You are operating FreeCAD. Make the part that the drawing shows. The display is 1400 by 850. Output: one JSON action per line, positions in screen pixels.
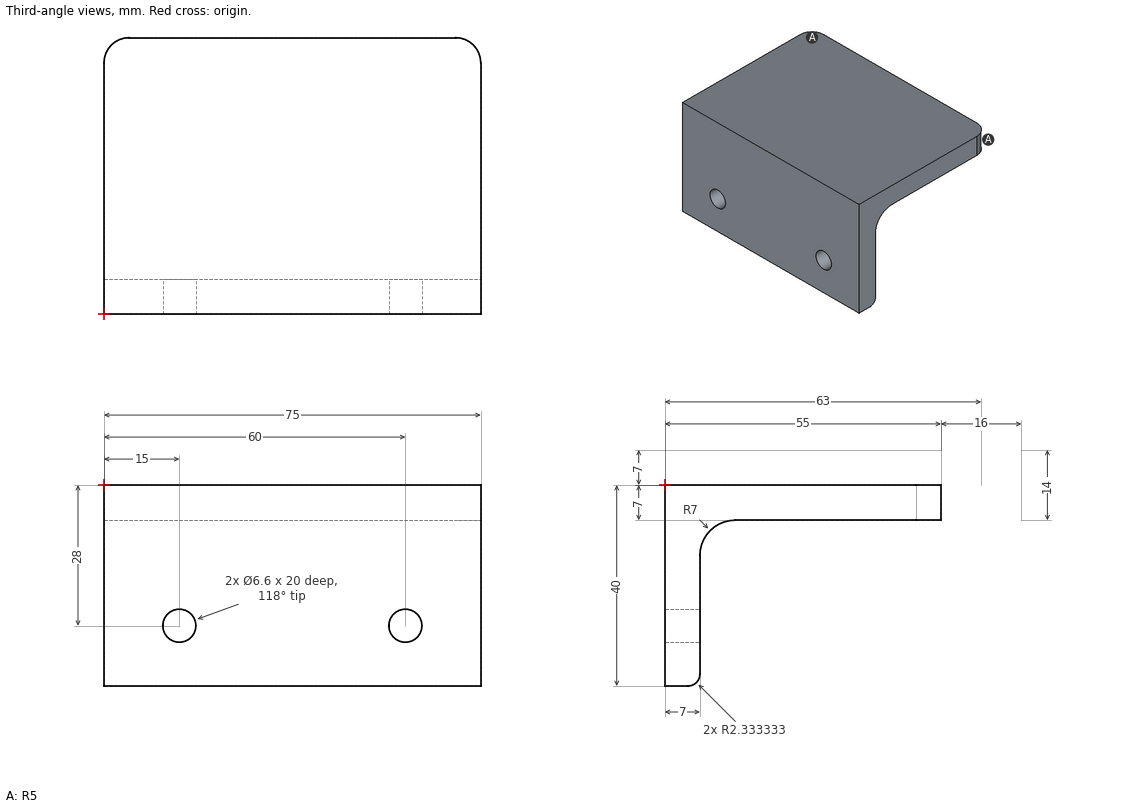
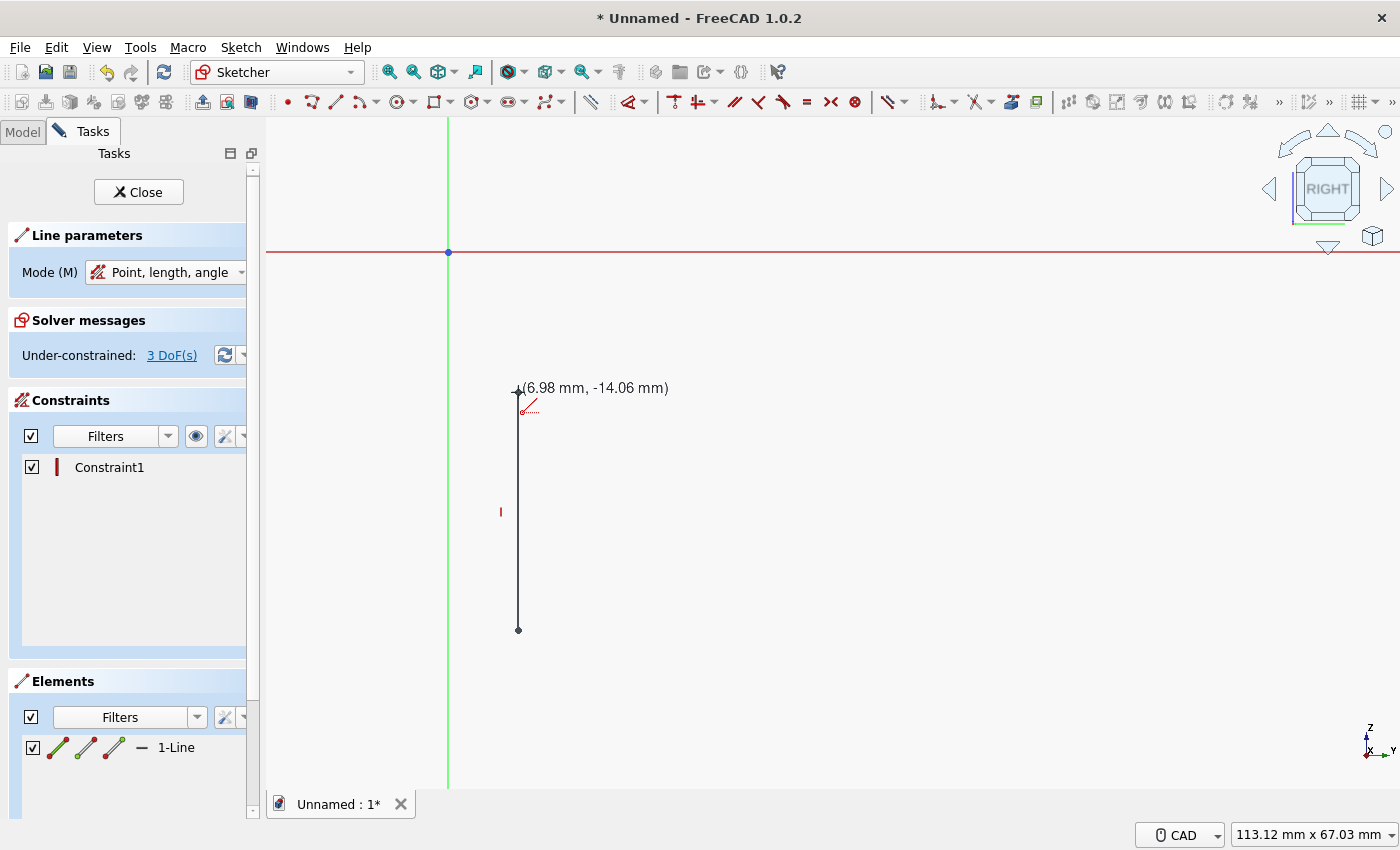
{"action": "left_click", "coordinate": [588, 322]}
{"action": "left_click", "coordinate": [1056, 322]}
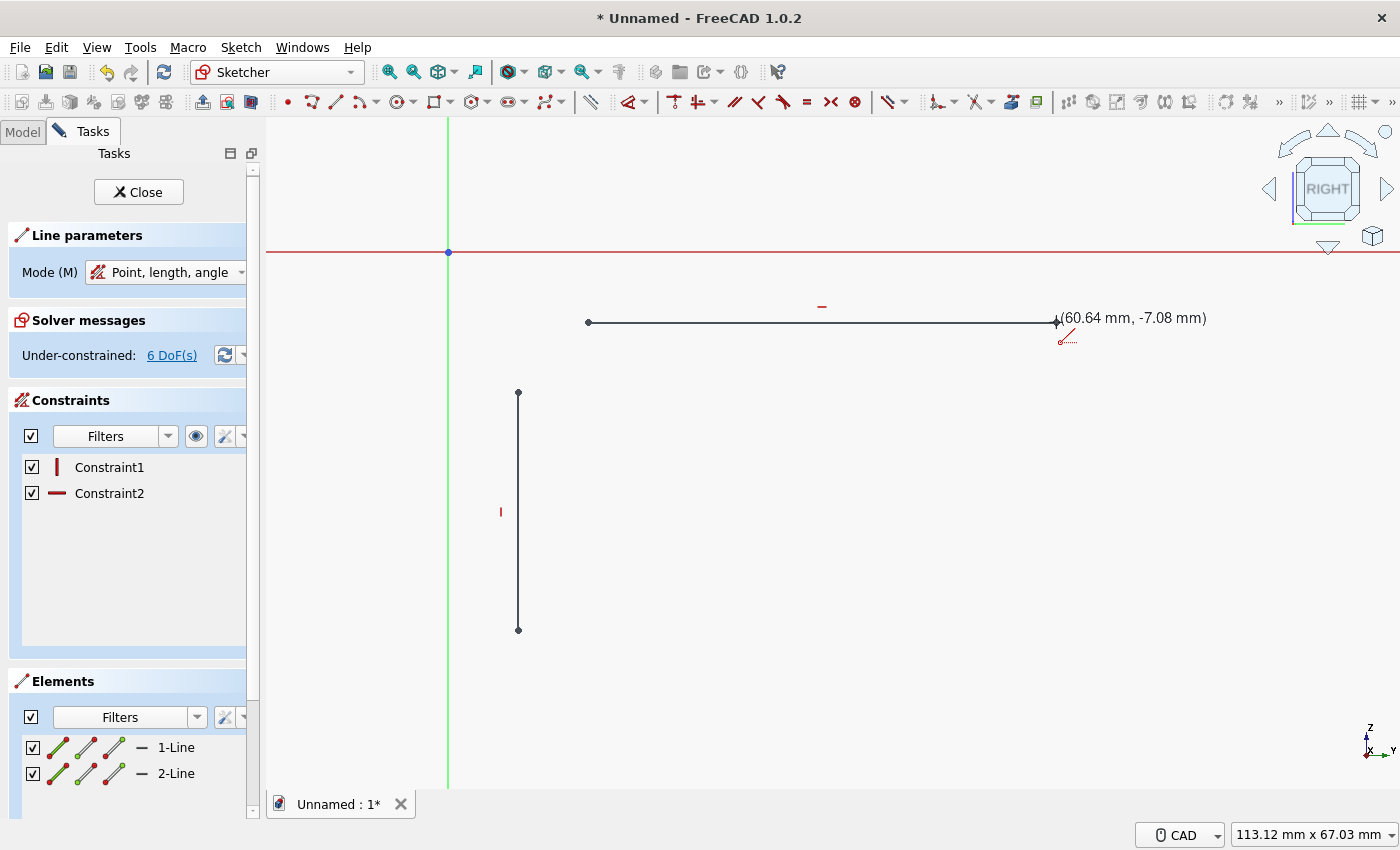
{"action": "left_click", "coordinate": [312, 102]}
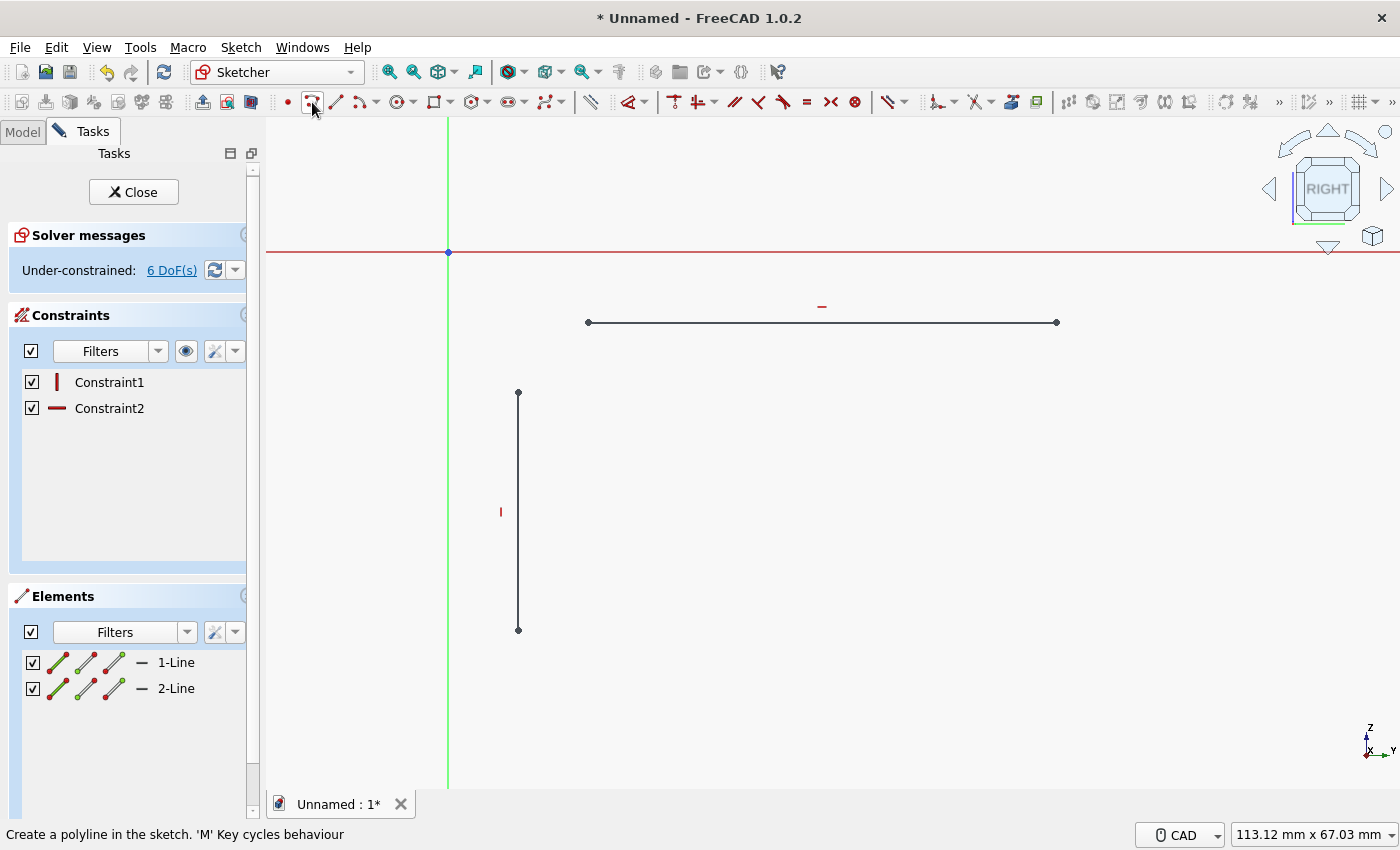
{"action": "left_click", "coordinate": [1080, 299]}
{"action": "left_click", "coordinate": [1080, 252]}
{"action": "left_click", "coordinate": [448, 252]}
{"action": "left_click", "coordinate": [457, 653]}
{"action": "left_click", "coordinate": [495, 653]}
{"action": "right_click", "coordinate": [495, 653]}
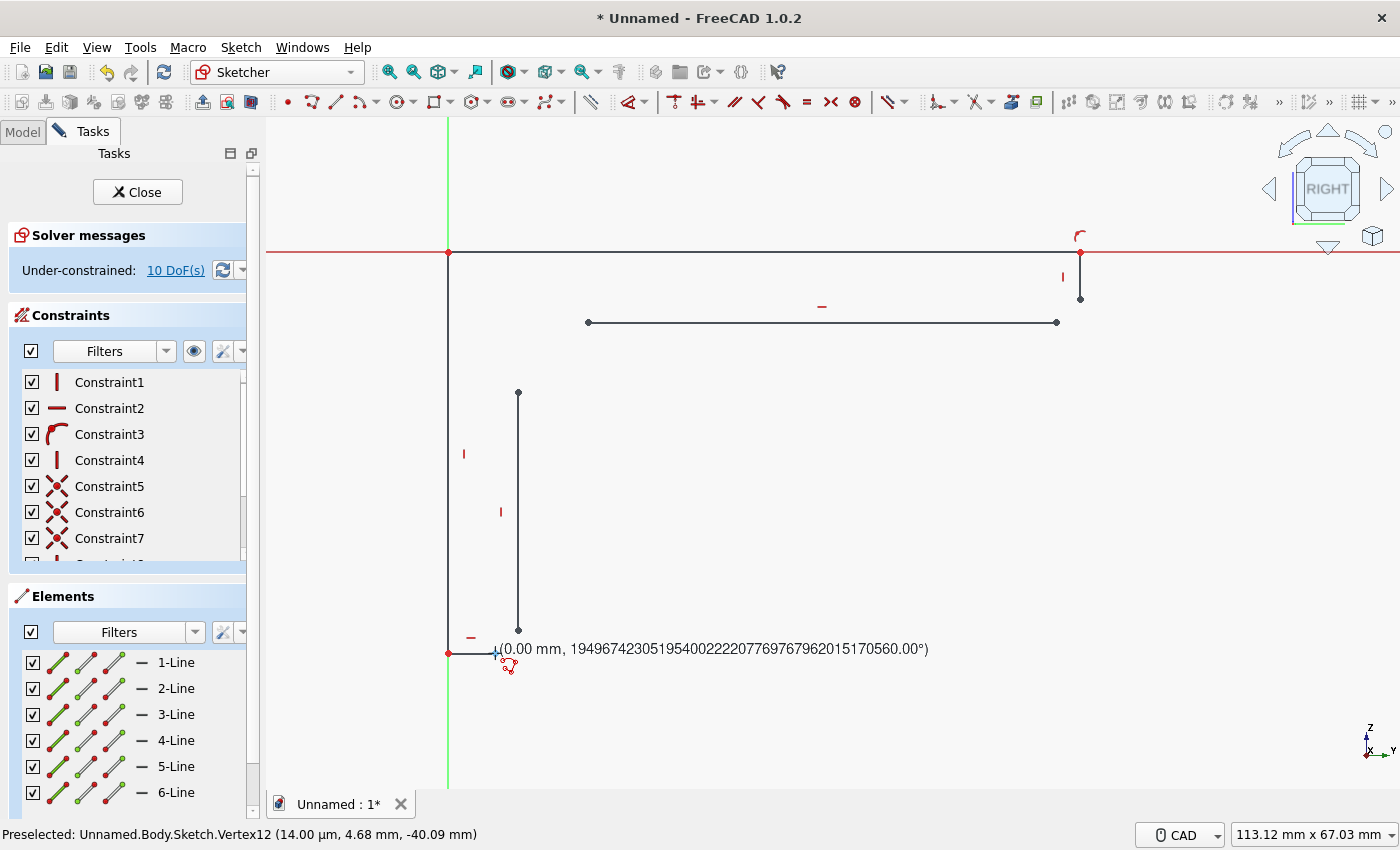
{"action": "left_click", "coordinate": [378, 102]}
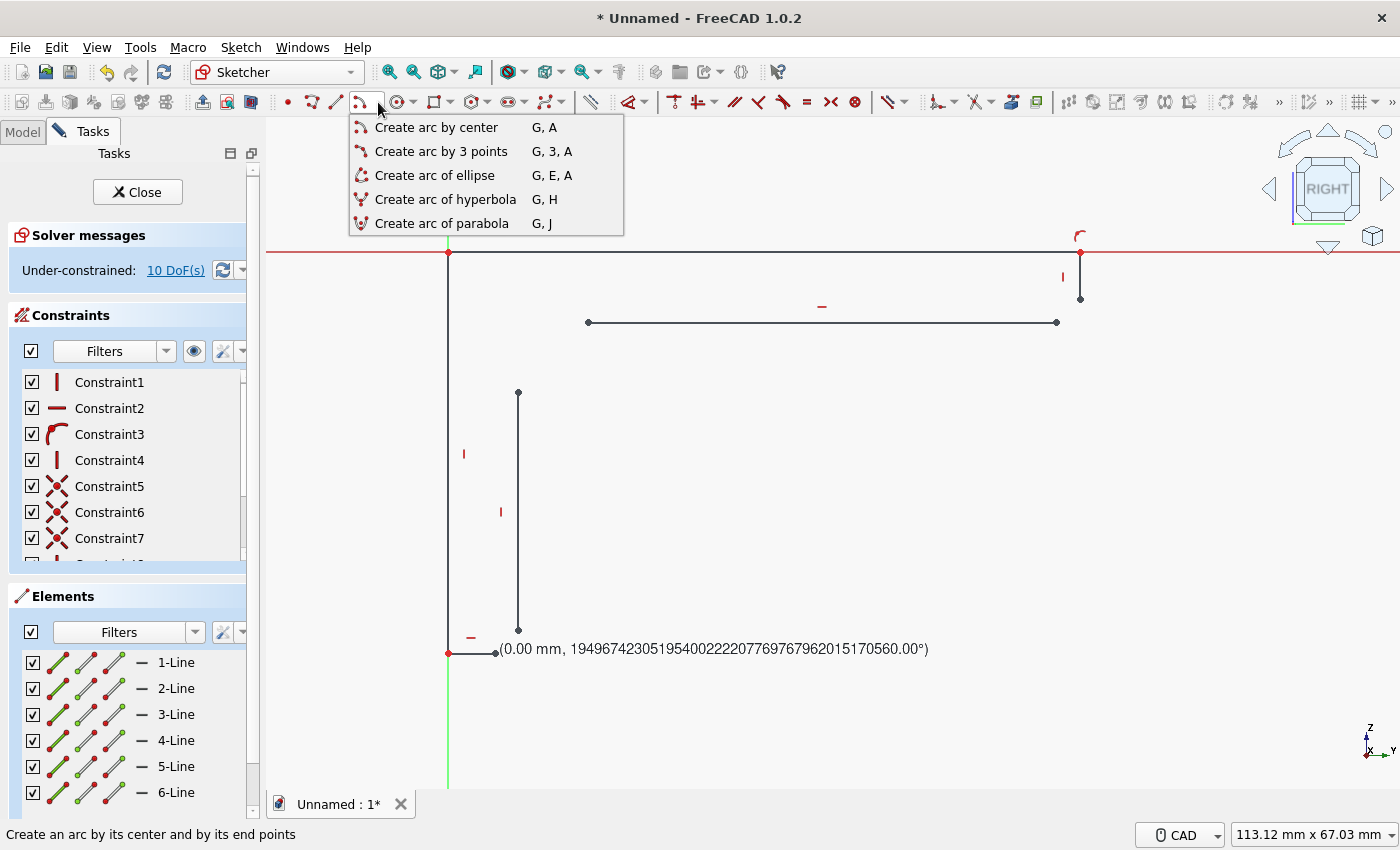
{"action": "left_click", "coordinate": [486, 151]}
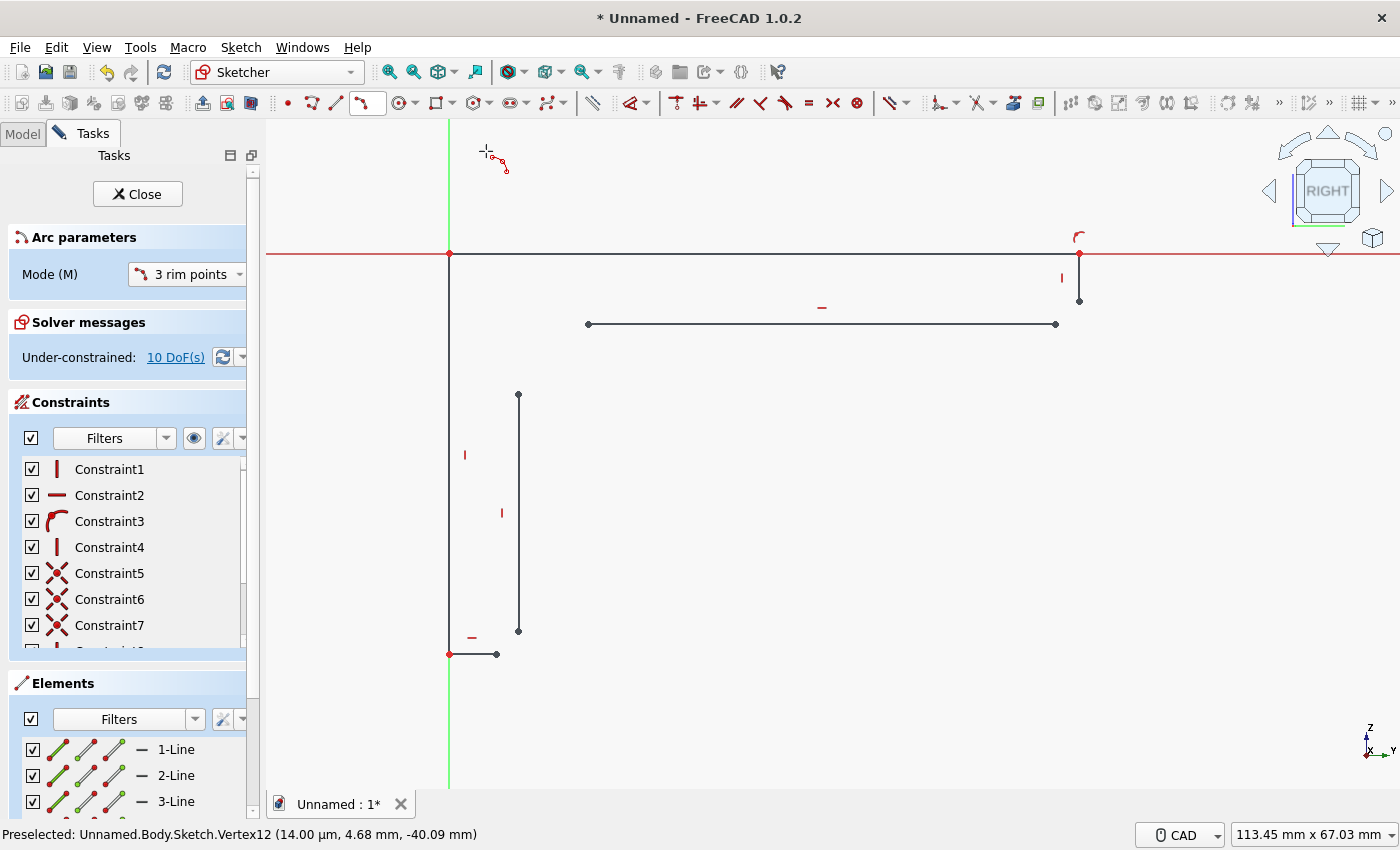
{"action": "left_click", "coordinate": [519, 394]}
{"action": "left_click", "coordinate": [589, 324]}
{"action": "left_click", "coordinate": [540, 344]}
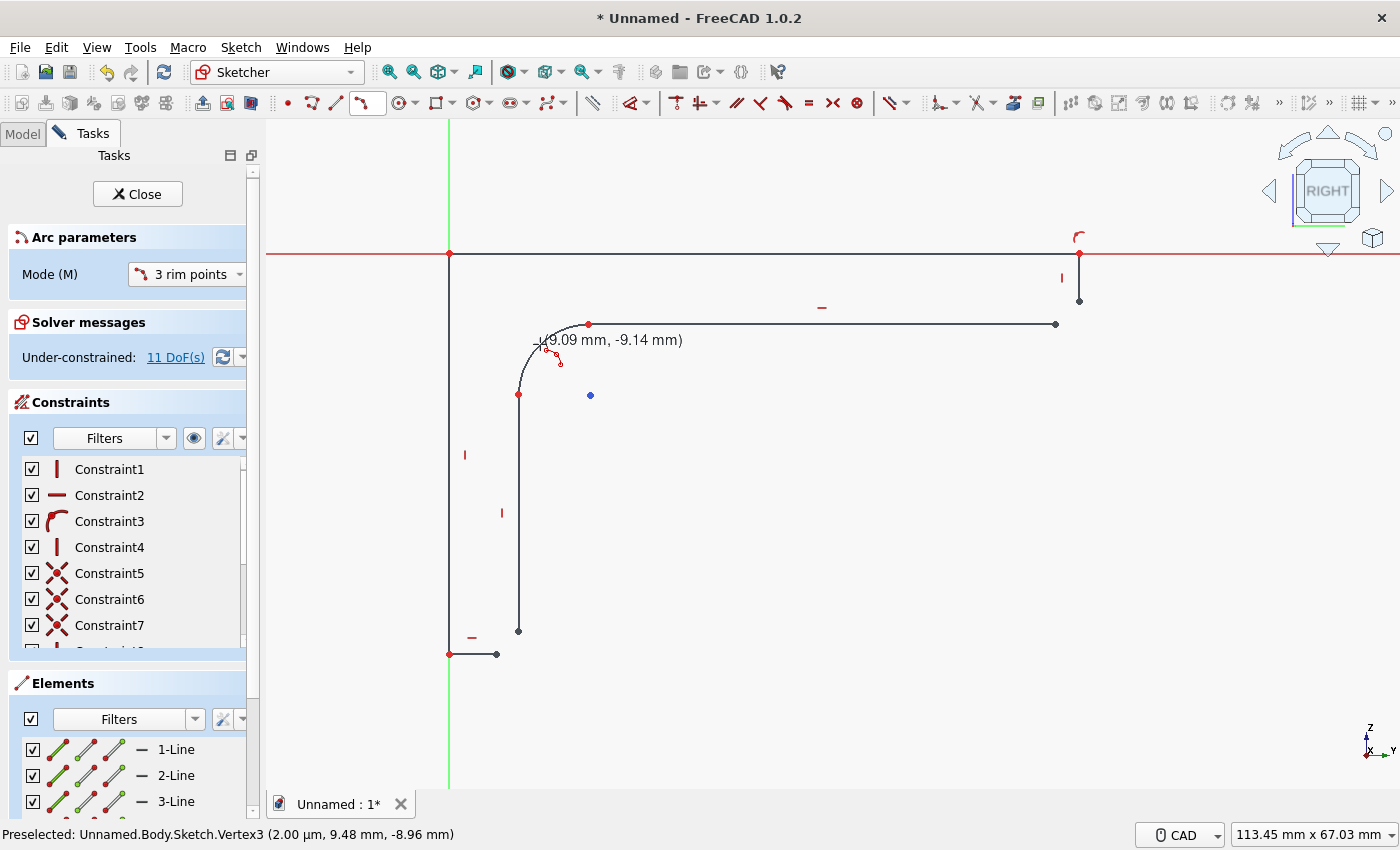
{"action": "left_click", "coordinate": [1055, 324]}
{"action": "left_click", "coordinate": [1079, 301]}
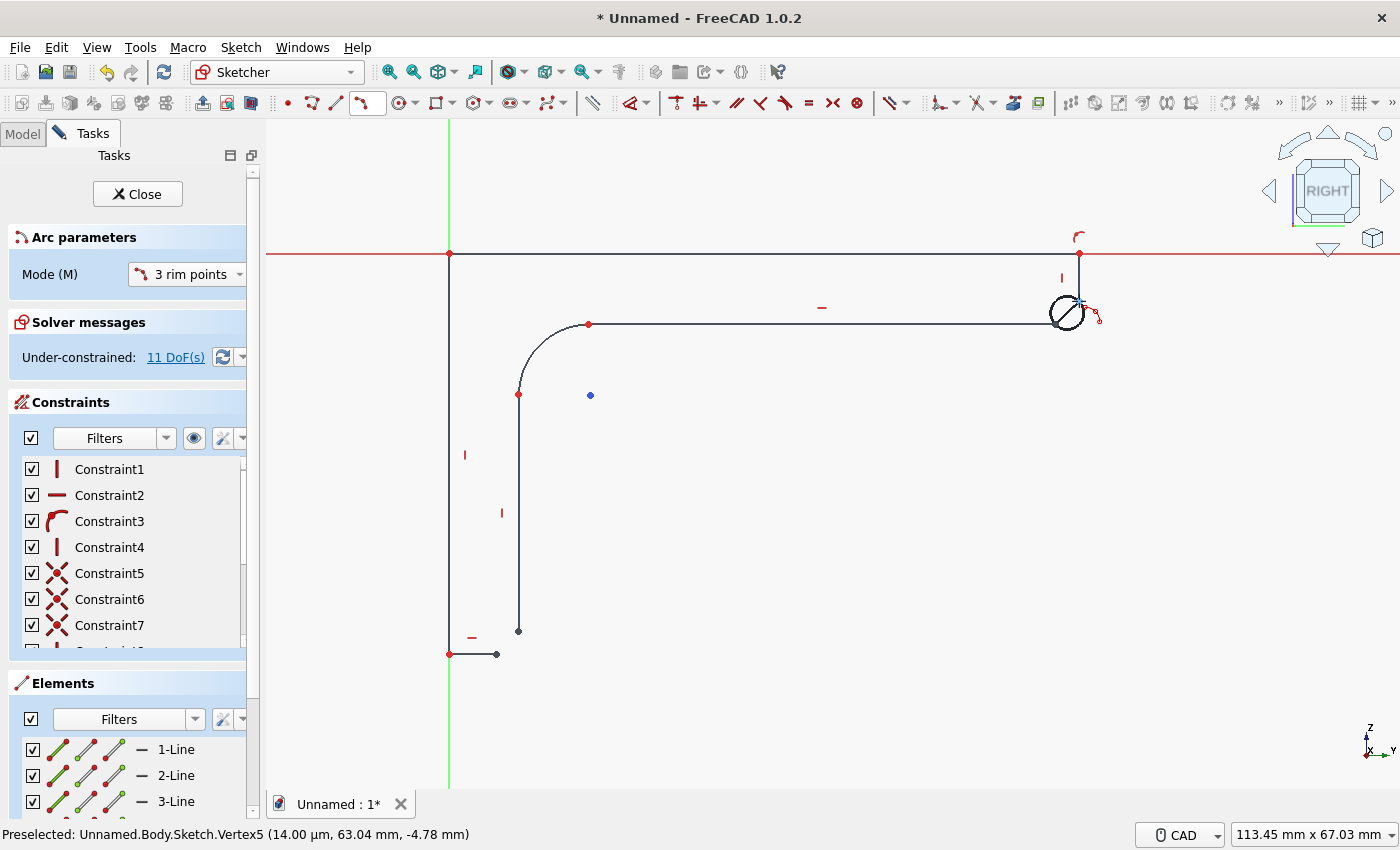
{"action": "scroll", "coordinate": [1072, 317], "scroll_direction": "up", "scroll_amount": 5}